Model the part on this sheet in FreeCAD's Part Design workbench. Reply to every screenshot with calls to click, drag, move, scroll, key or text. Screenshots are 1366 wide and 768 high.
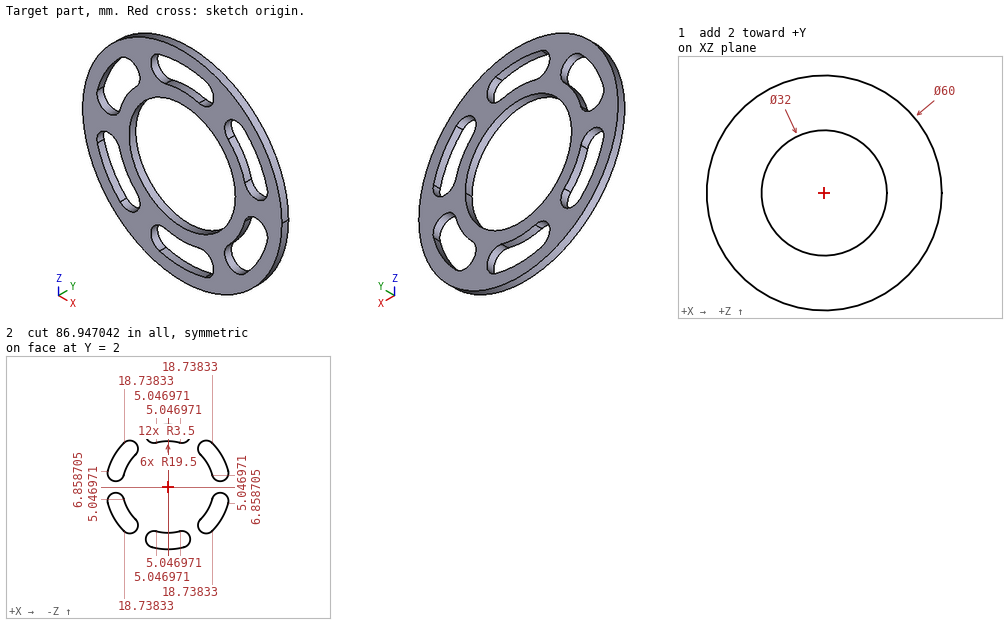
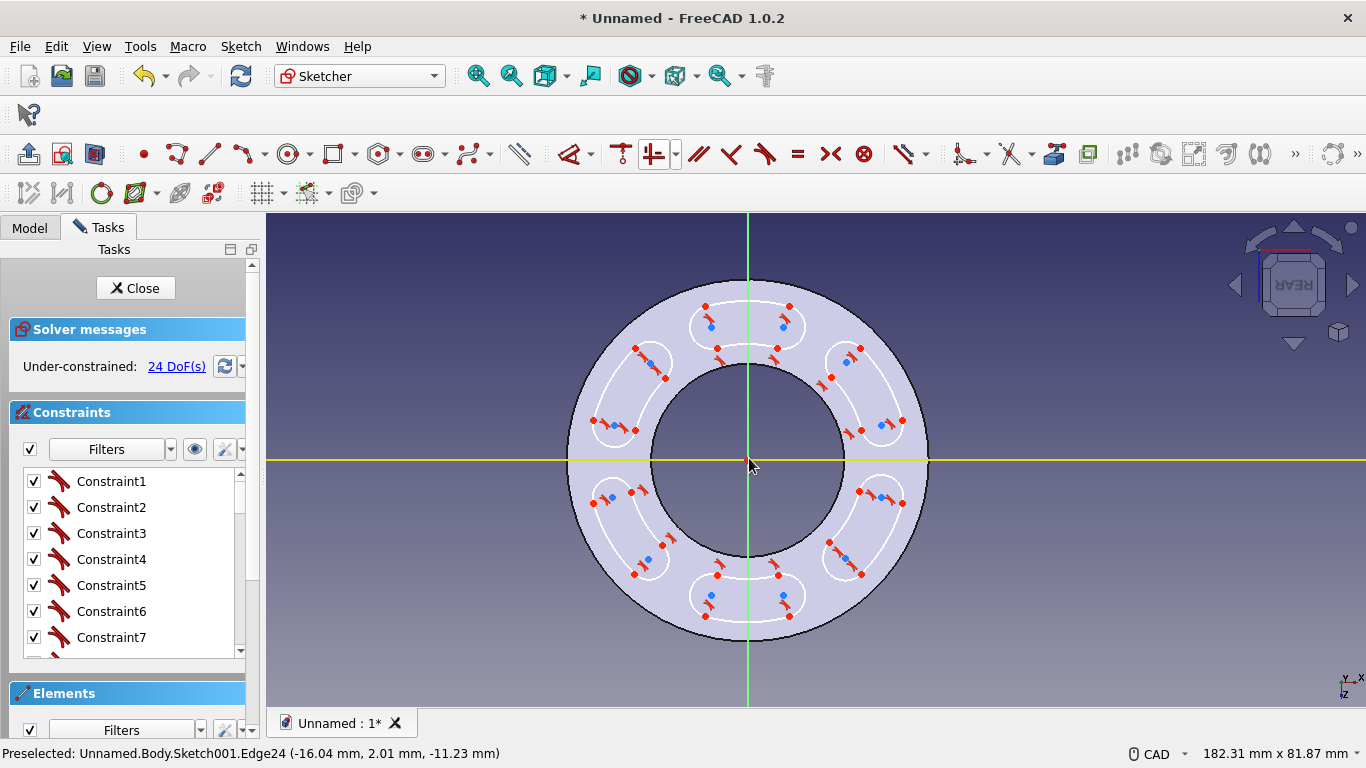
click(760, 345)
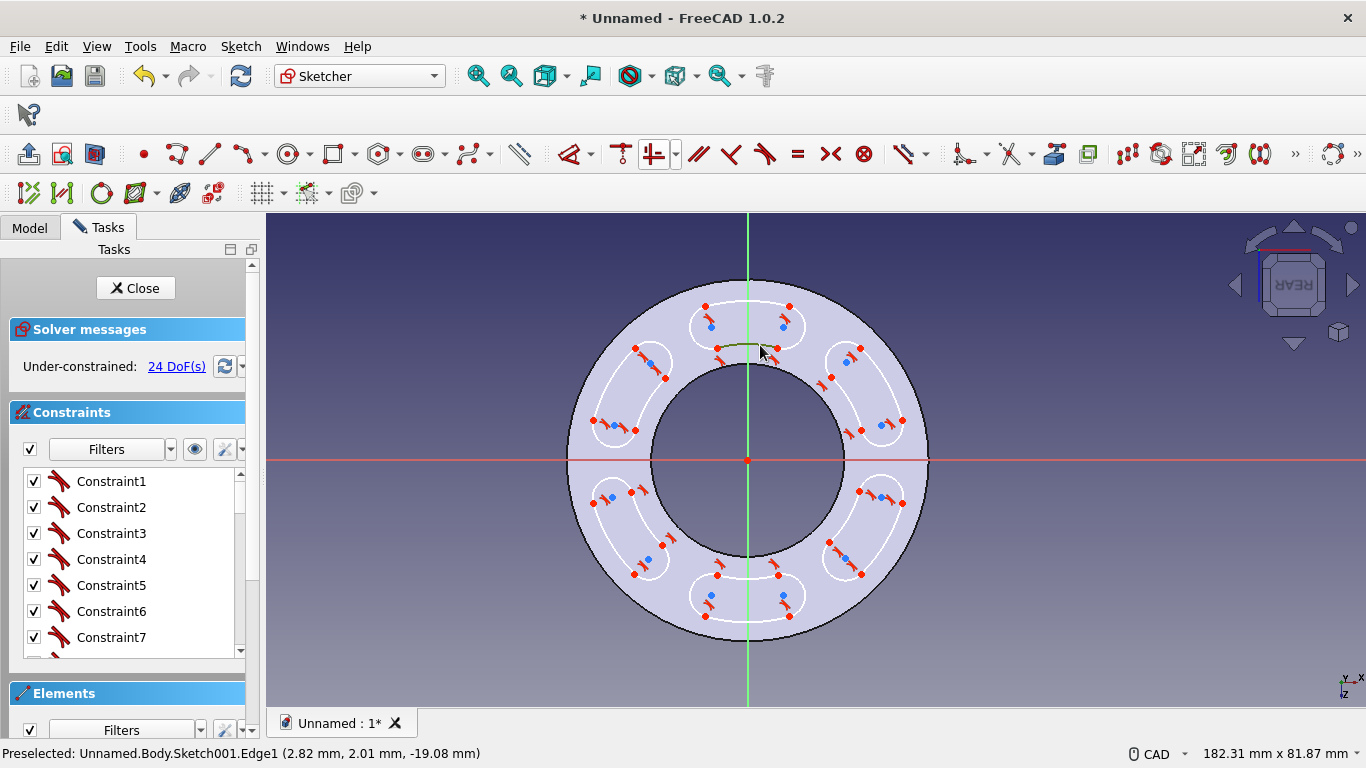
click(856, 413)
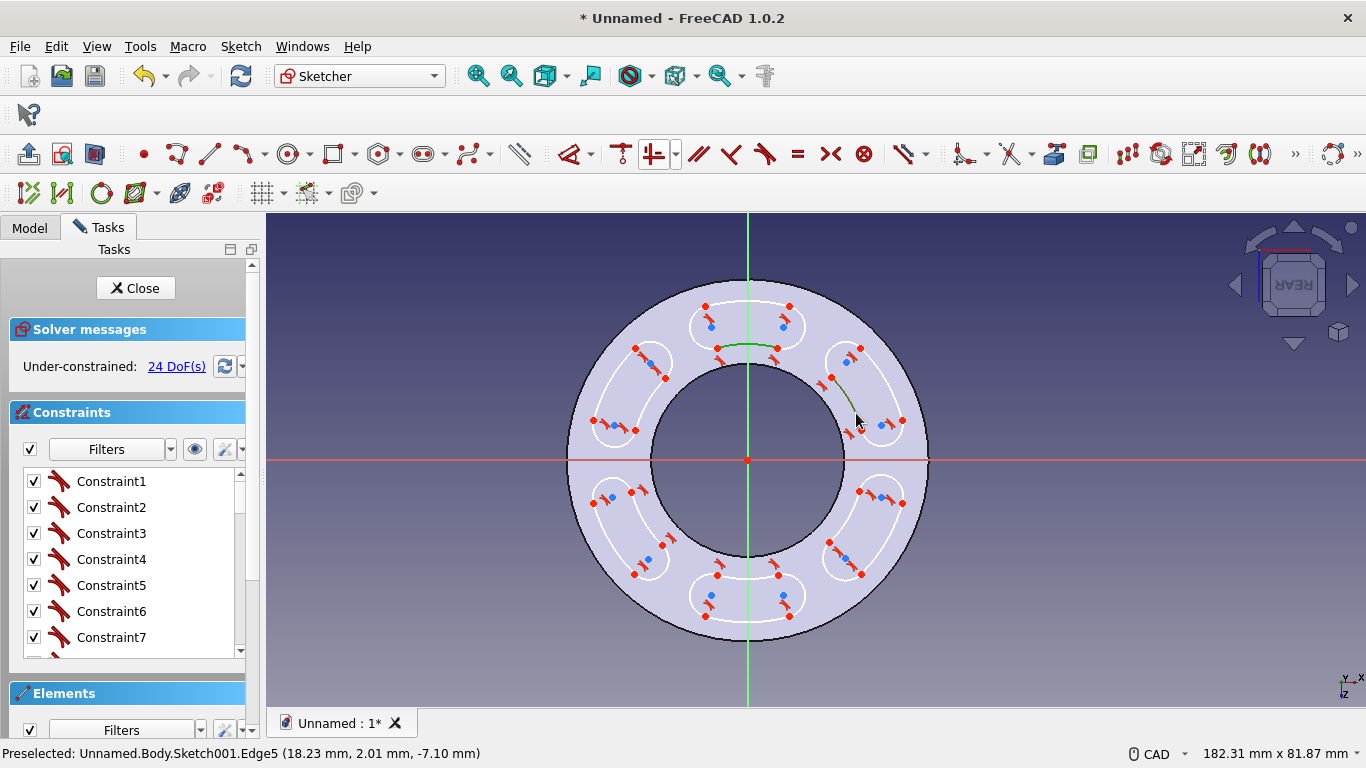
click(841, 529)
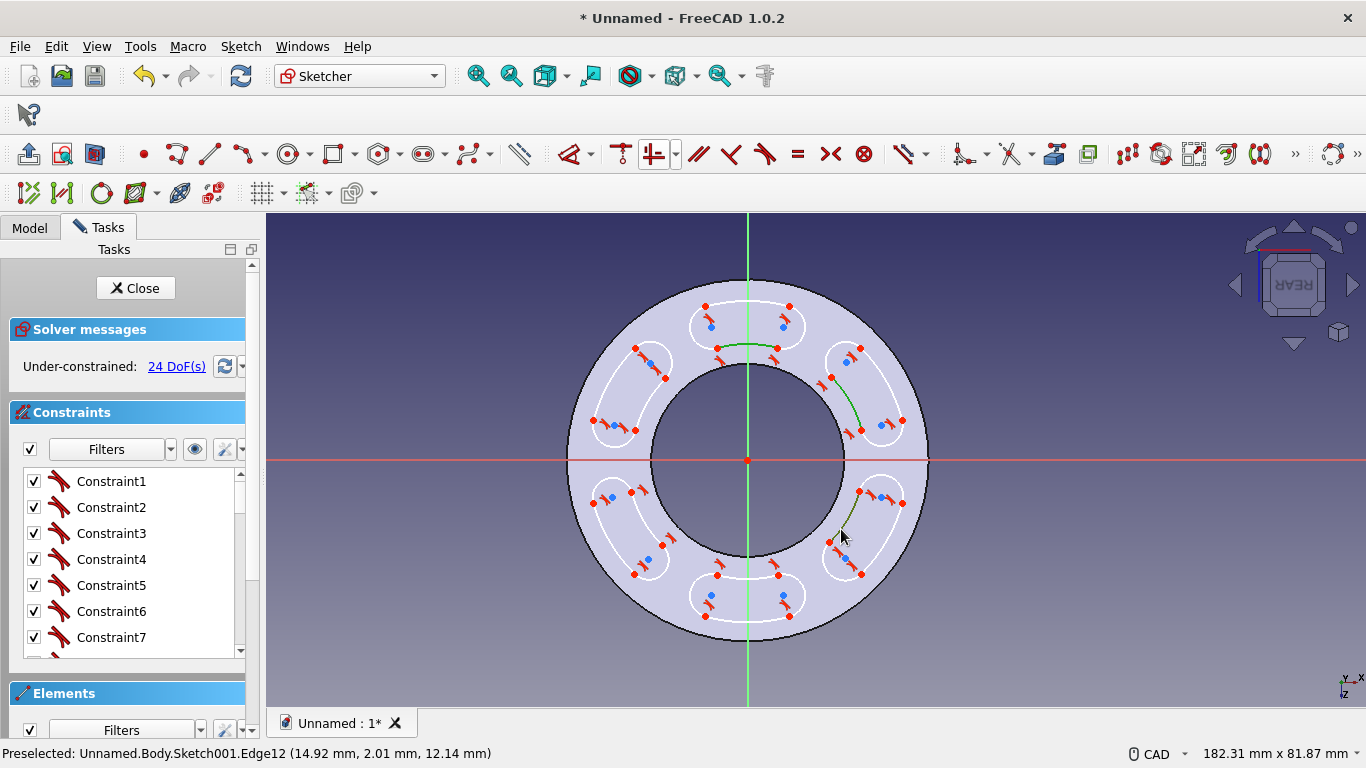
click(735, 578)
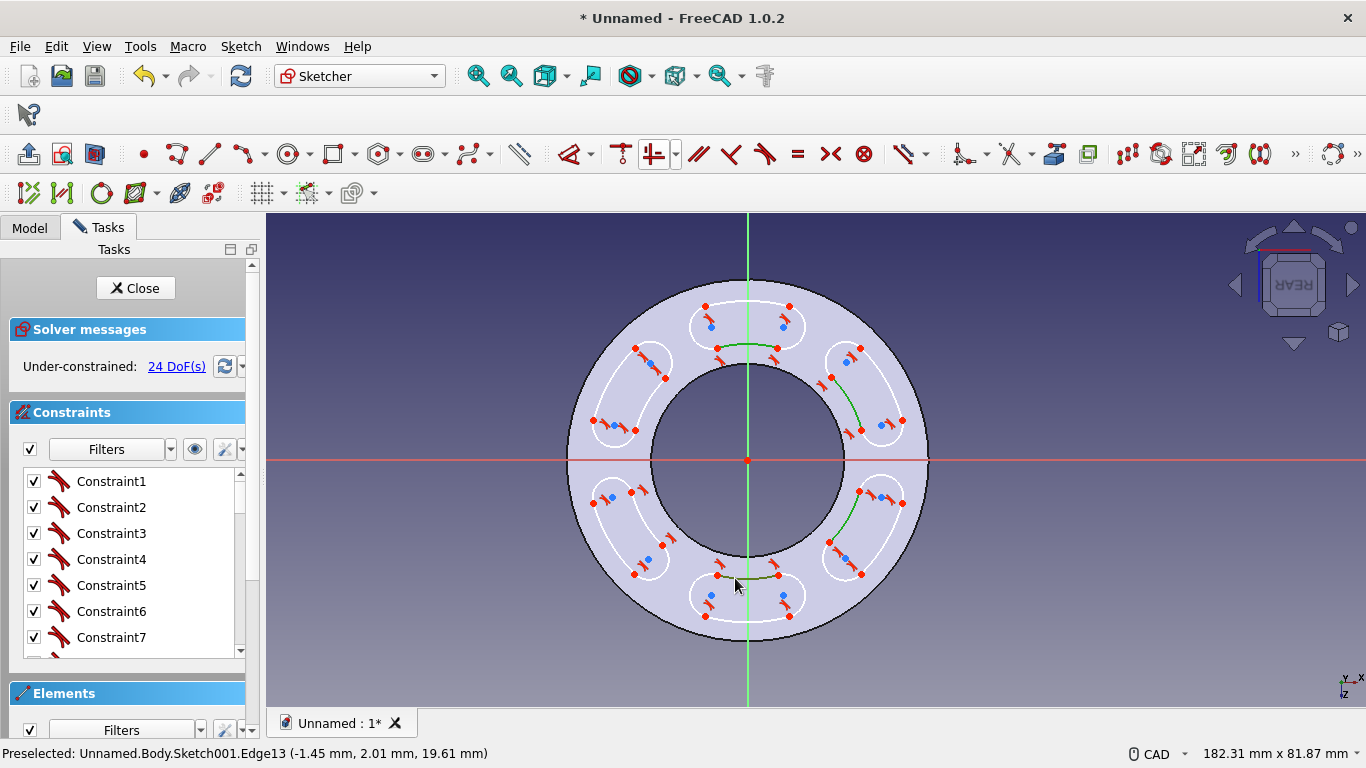
click(638, 510)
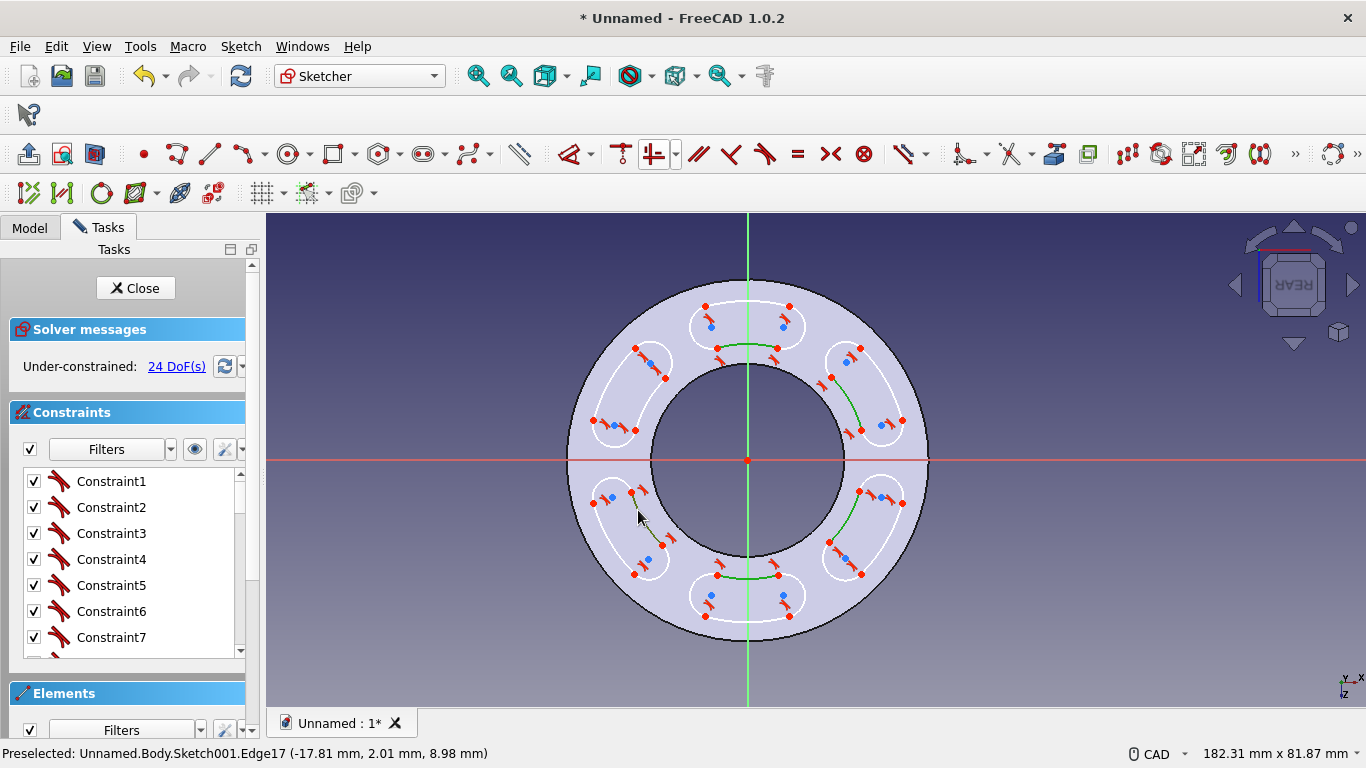
click(654, 393)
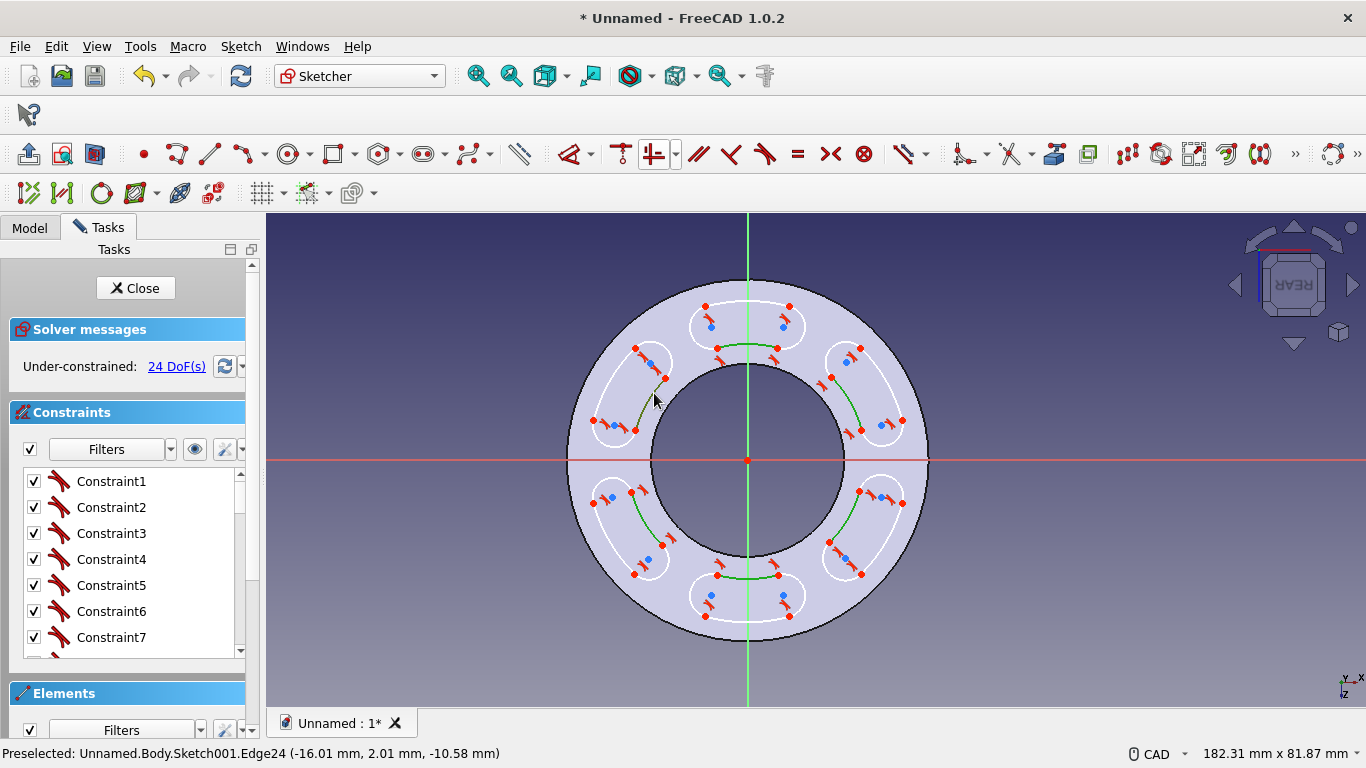
click(798, 154)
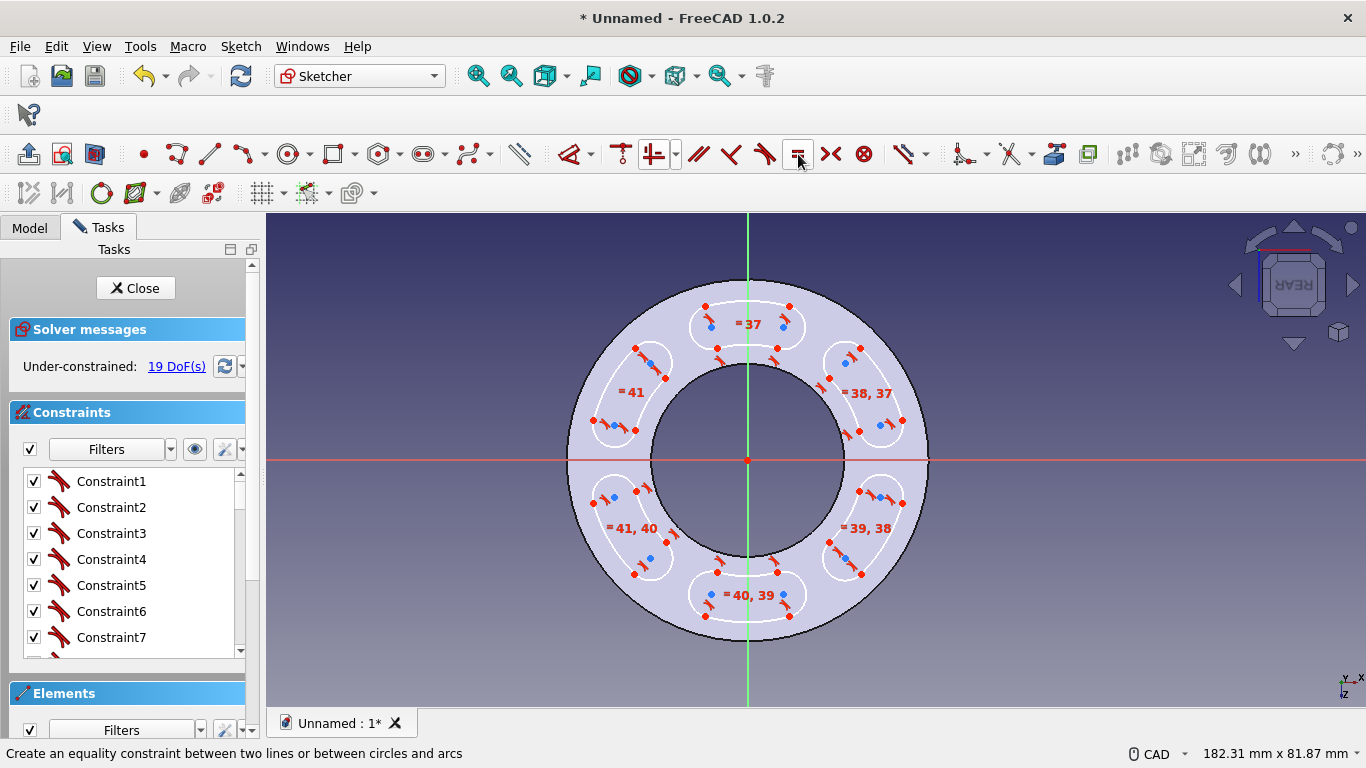
click(797, 345)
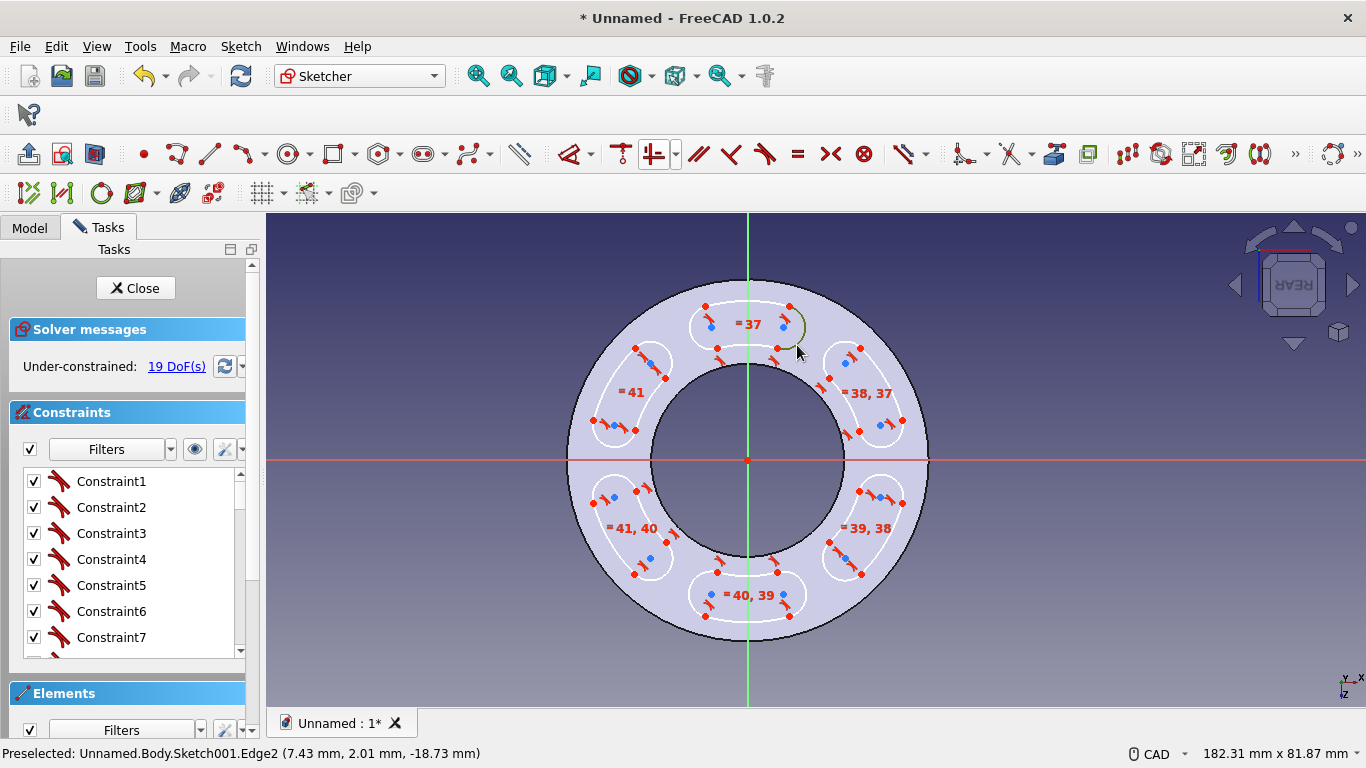
click(873, 446)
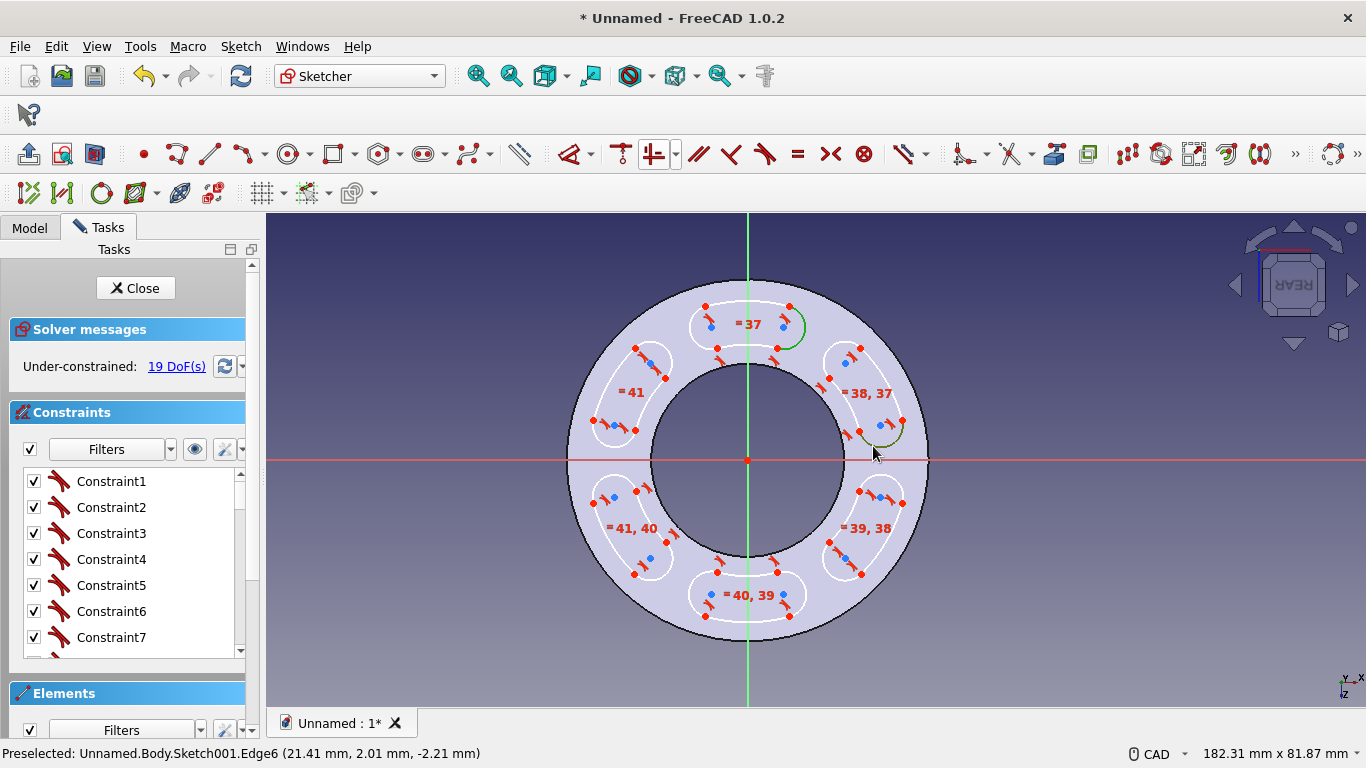
click(823, 562)